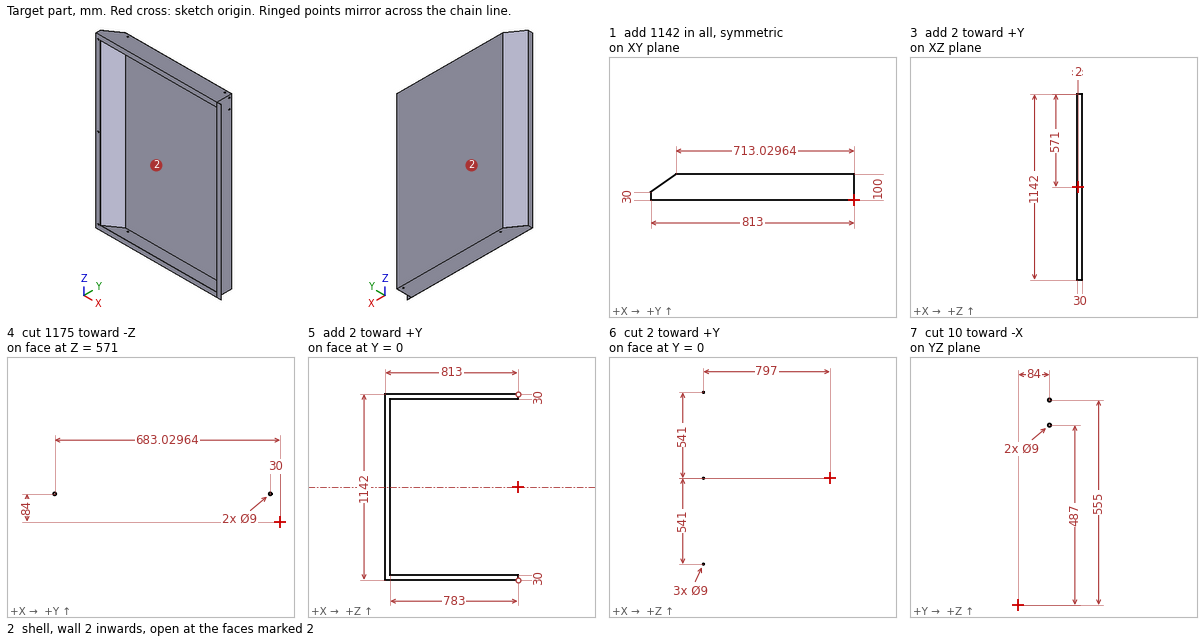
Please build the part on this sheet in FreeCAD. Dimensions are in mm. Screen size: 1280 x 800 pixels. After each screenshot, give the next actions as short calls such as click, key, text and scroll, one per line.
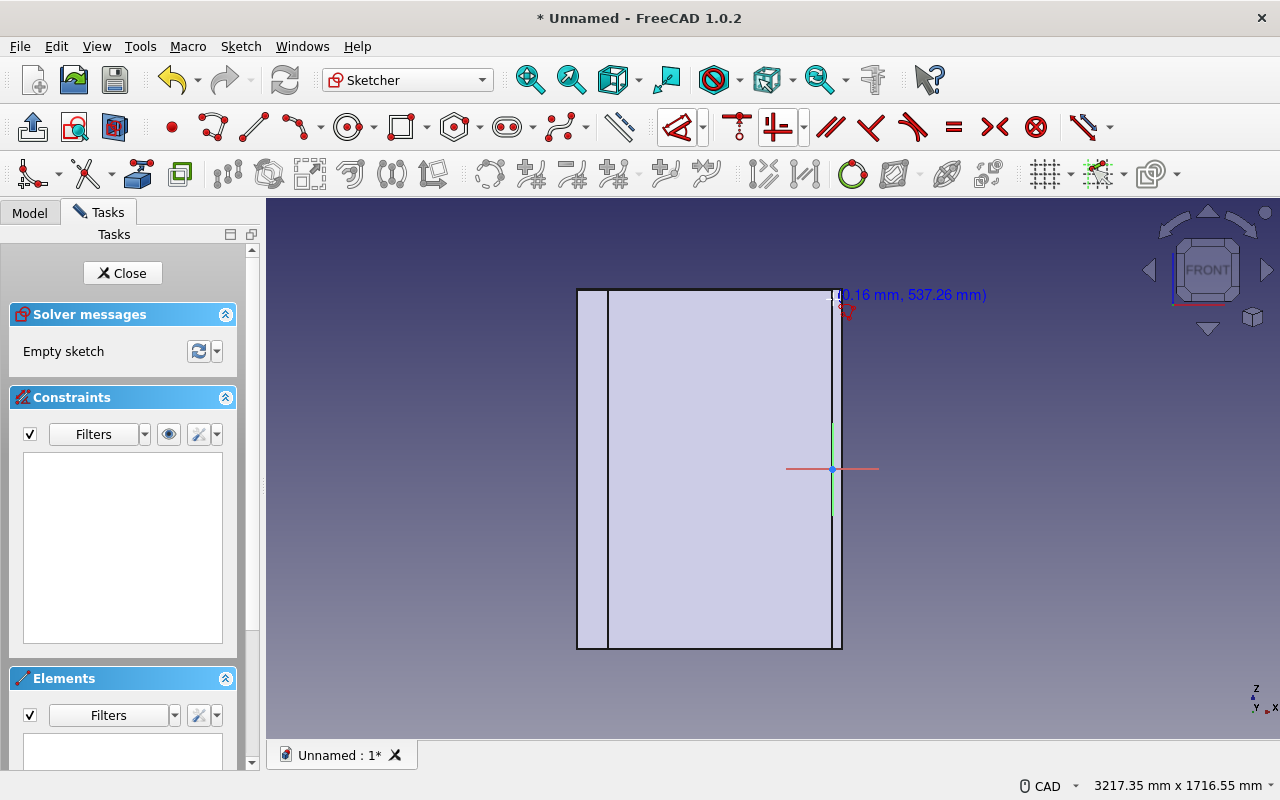
scroll(833, 289, up, 3)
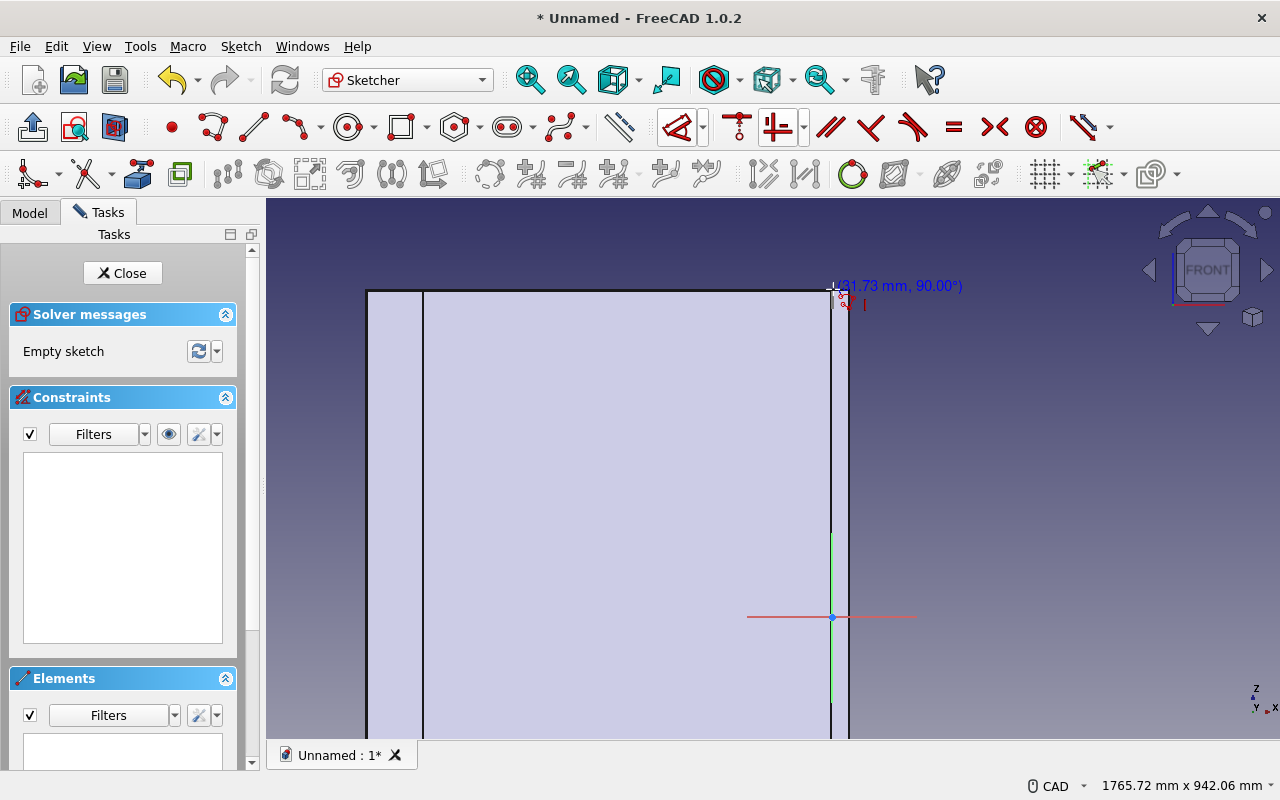
click(823, 290)
click(366, 290)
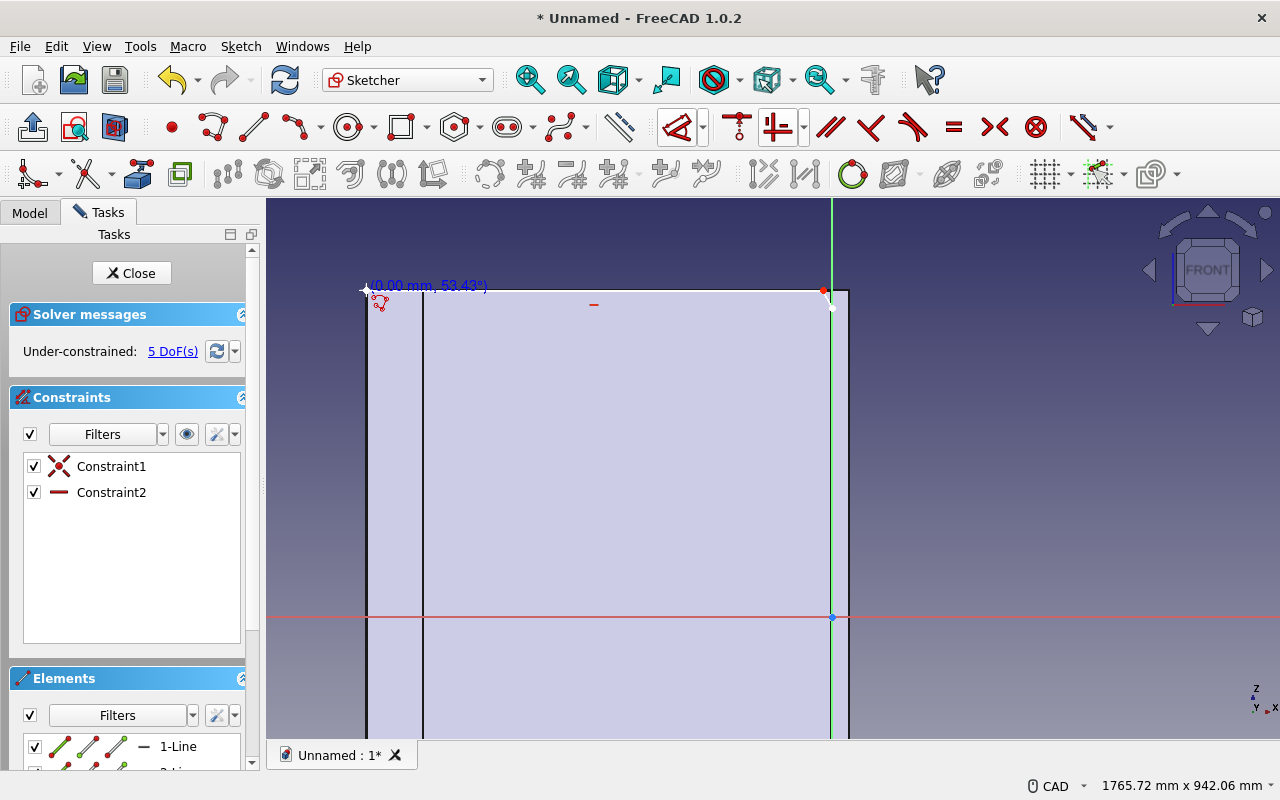
scroll(833, 287, down, 3)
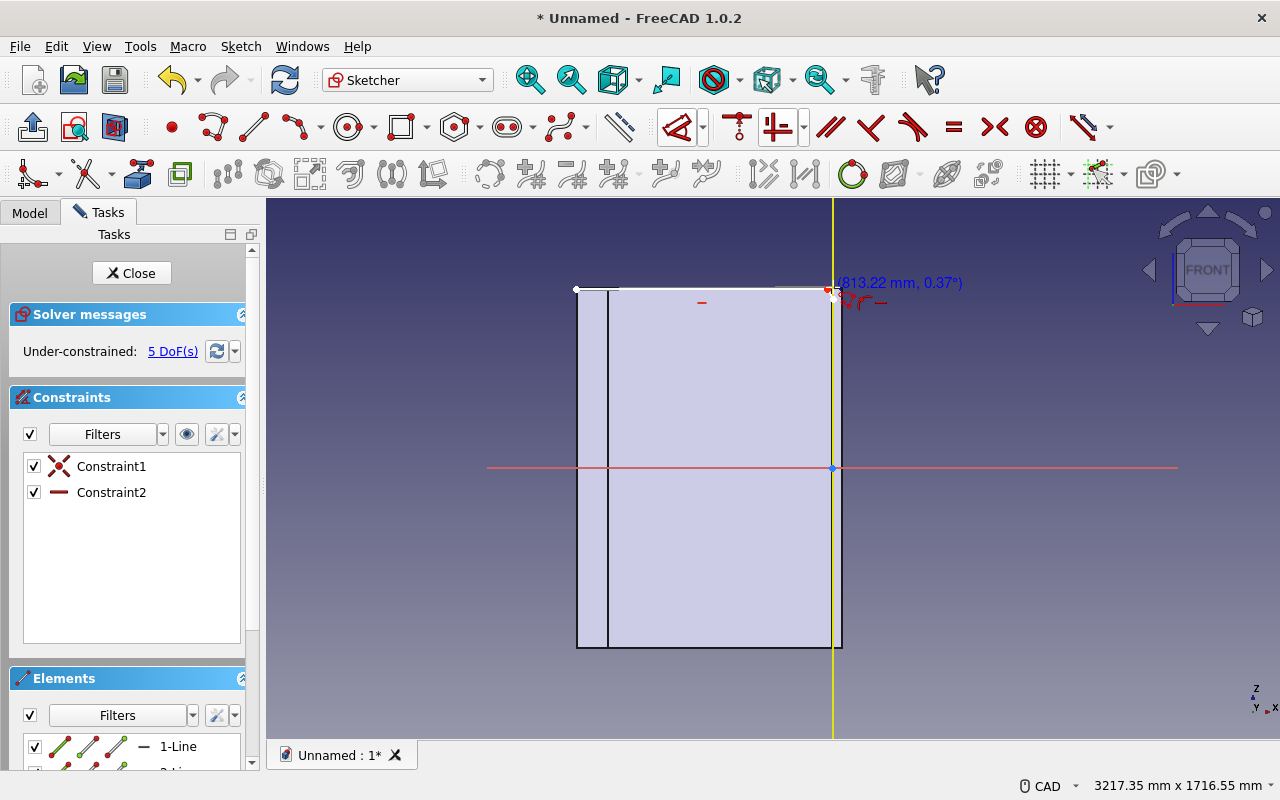
click(577, 648)
click(833, 648)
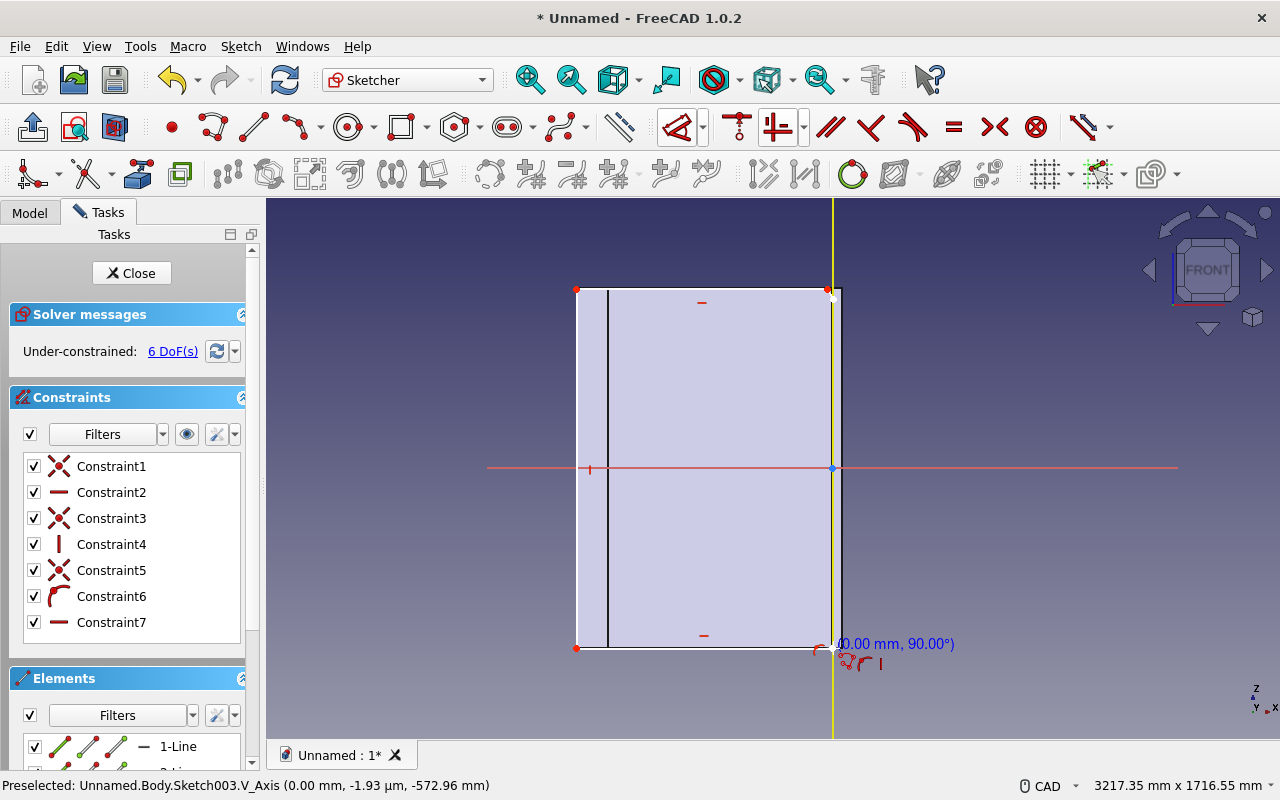
scroll(833, 639, up, 3)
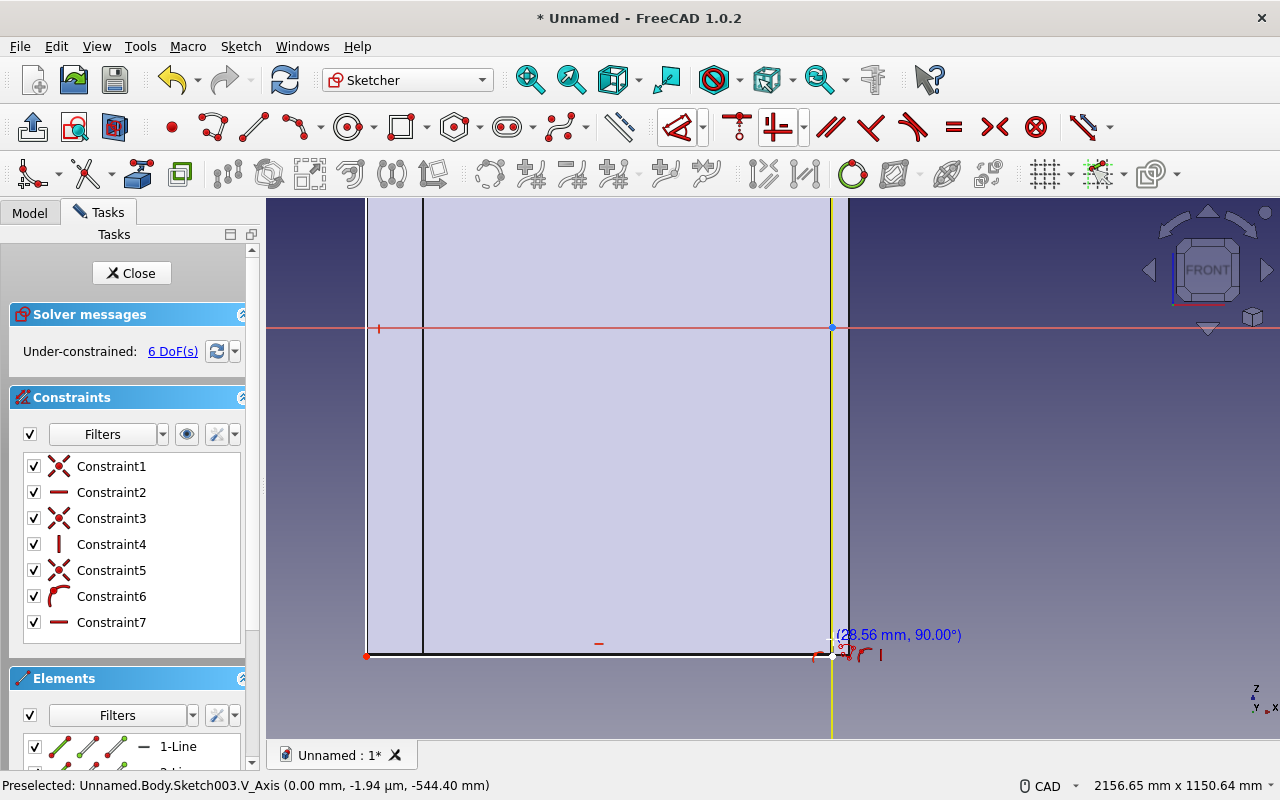
click(823, 638)
click(383, 638)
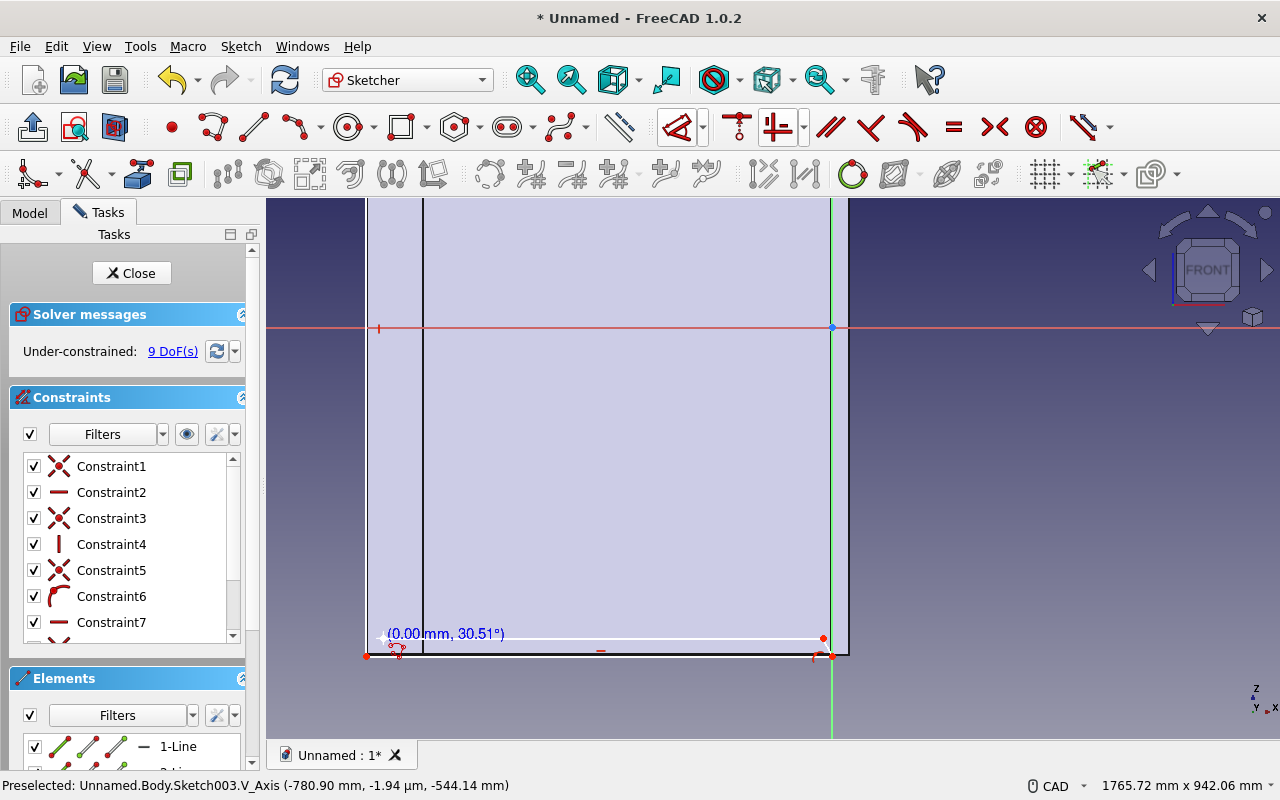
scroll(833, 640, down, 3)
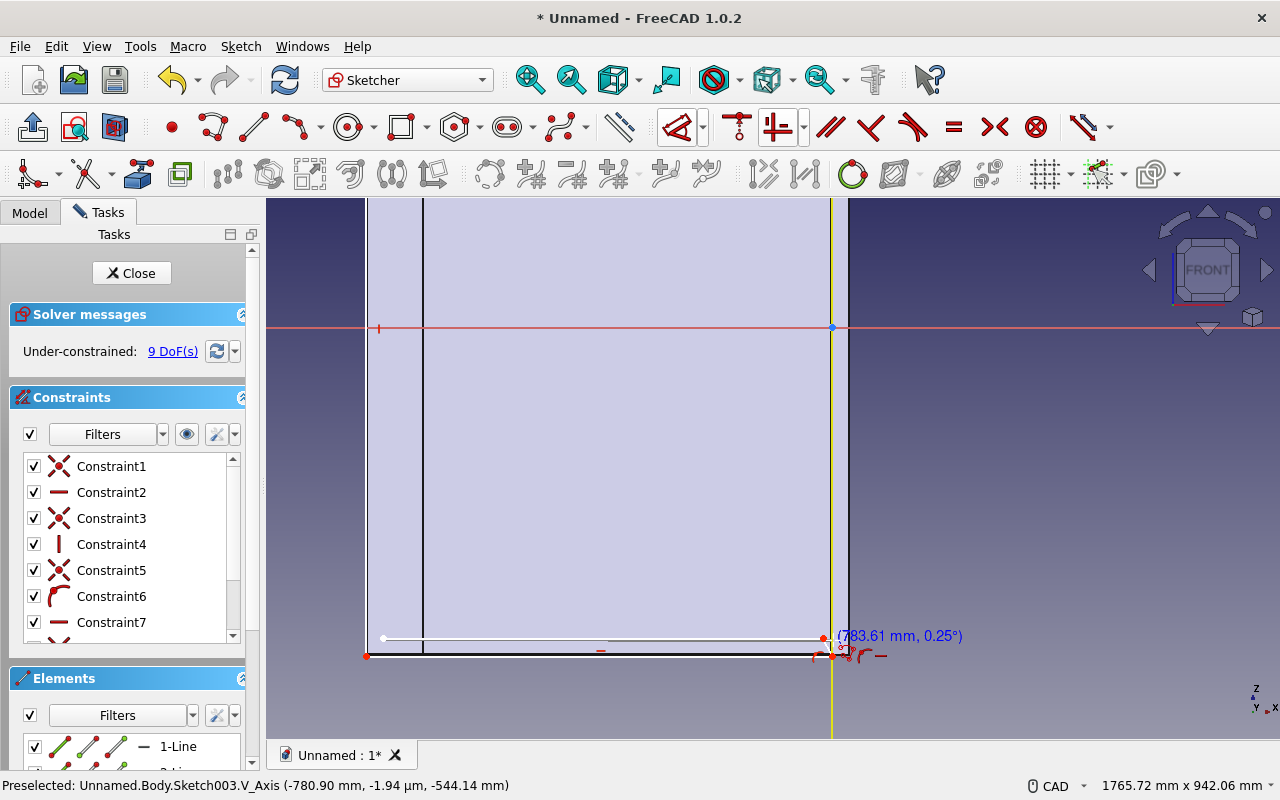
scroll(586, 298, up, 3)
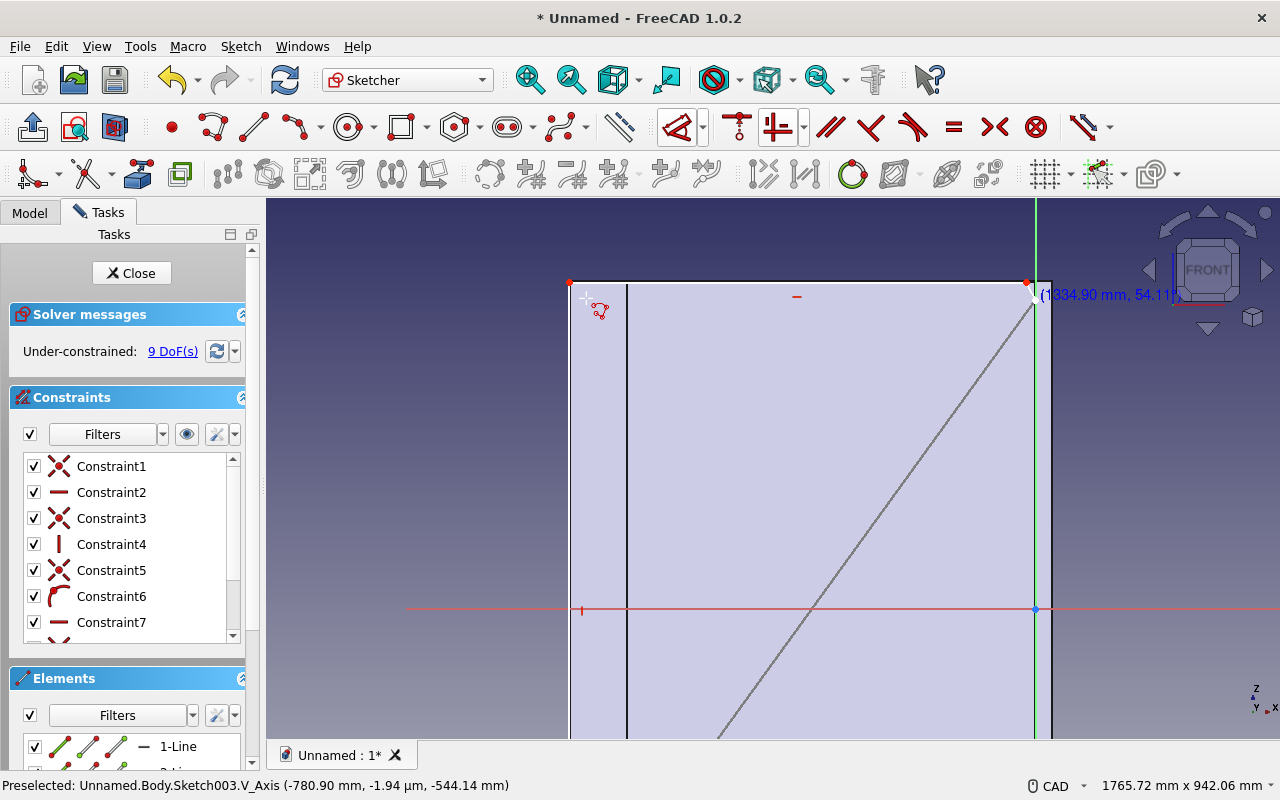
click(586, 299)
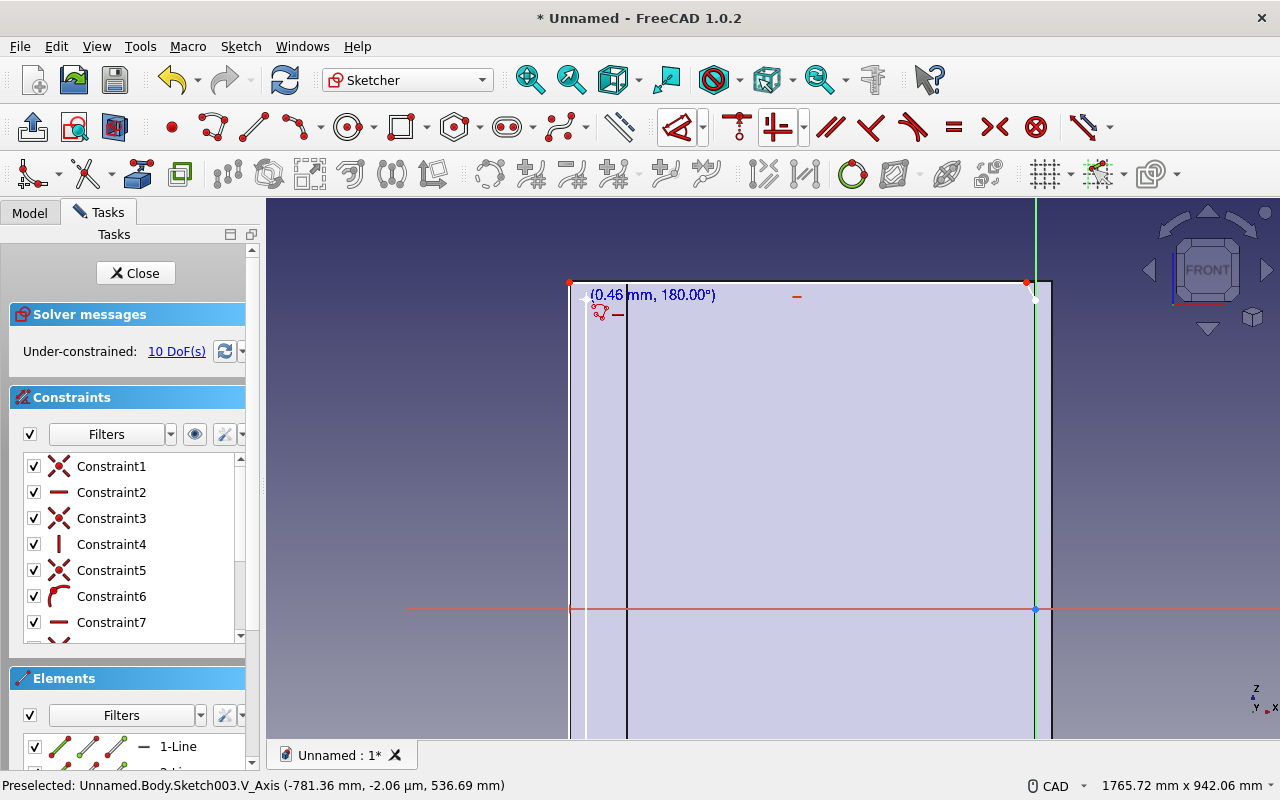
scroll(1036, 299, up, 4)